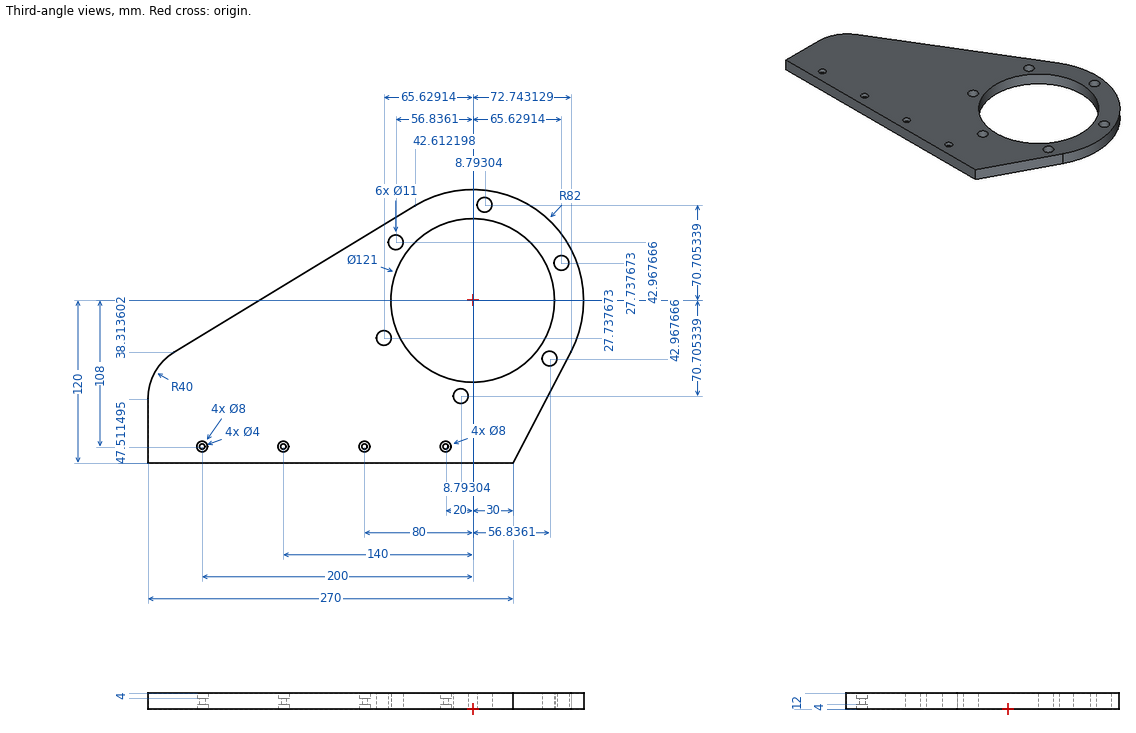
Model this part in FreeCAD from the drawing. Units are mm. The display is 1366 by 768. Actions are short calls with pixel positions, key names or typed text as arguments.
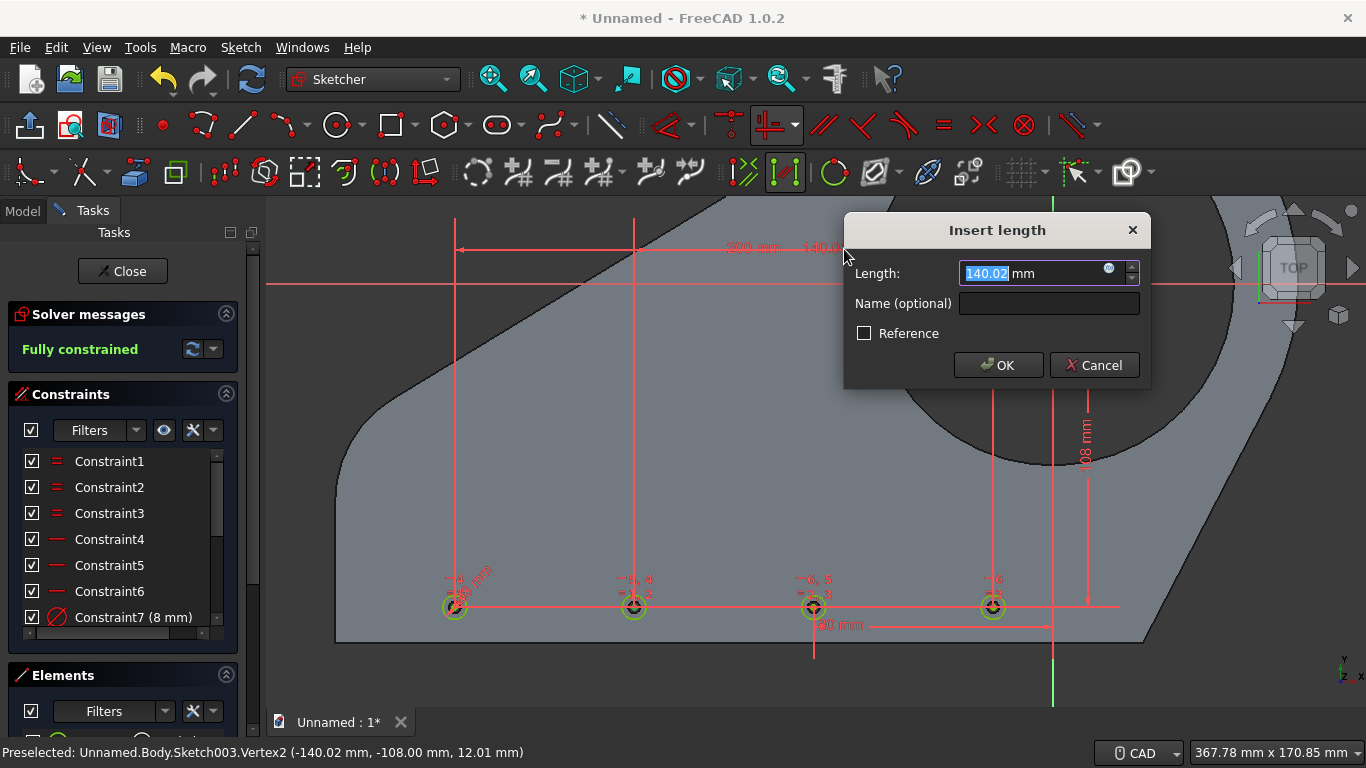
text(140)
key(Return)
key(Escape)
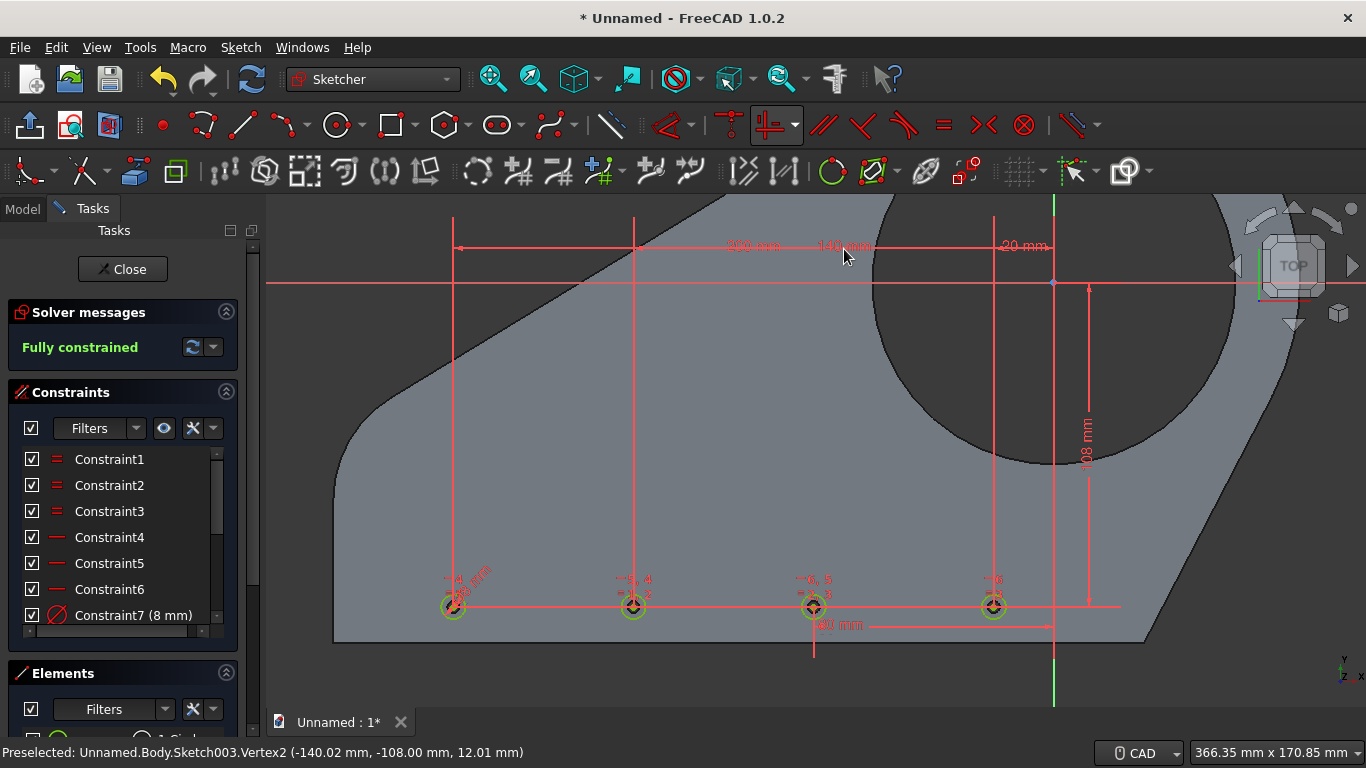
click(123, 269)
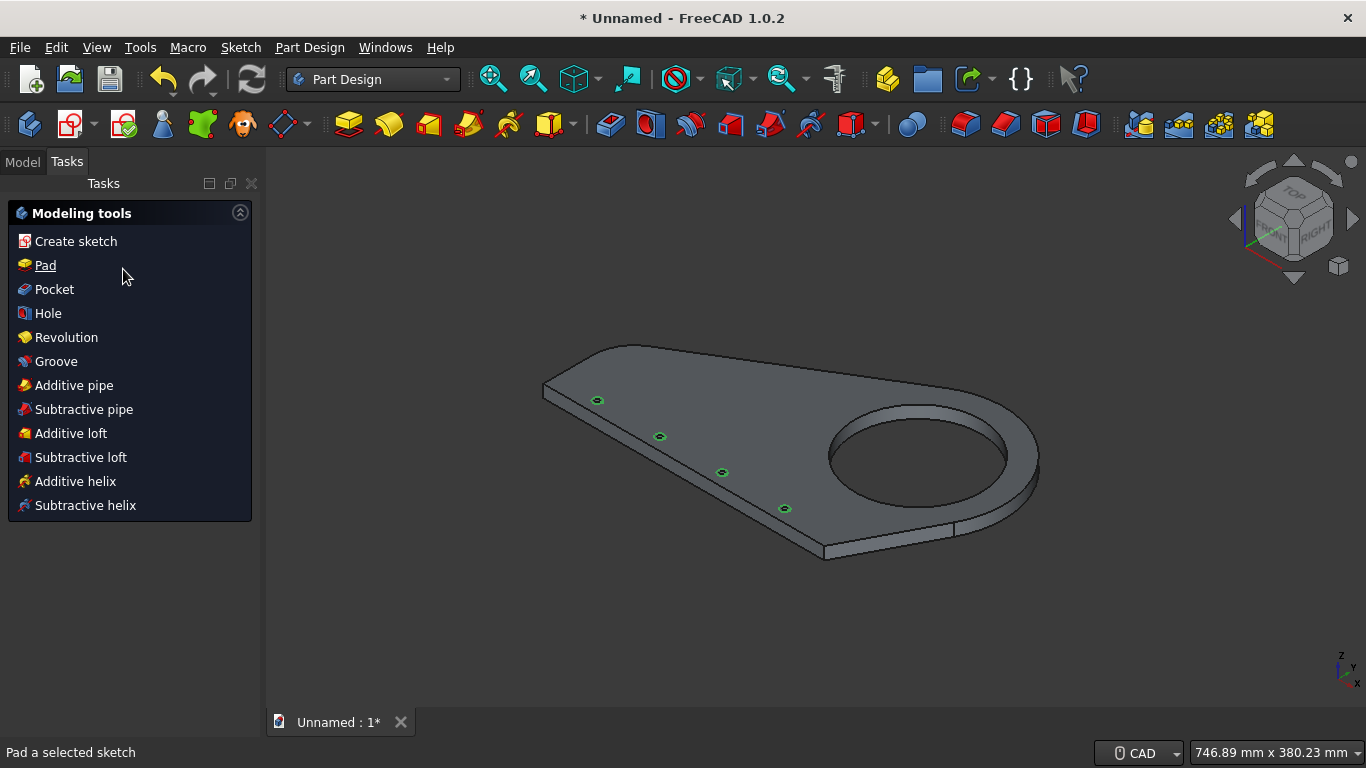
click(612, 124)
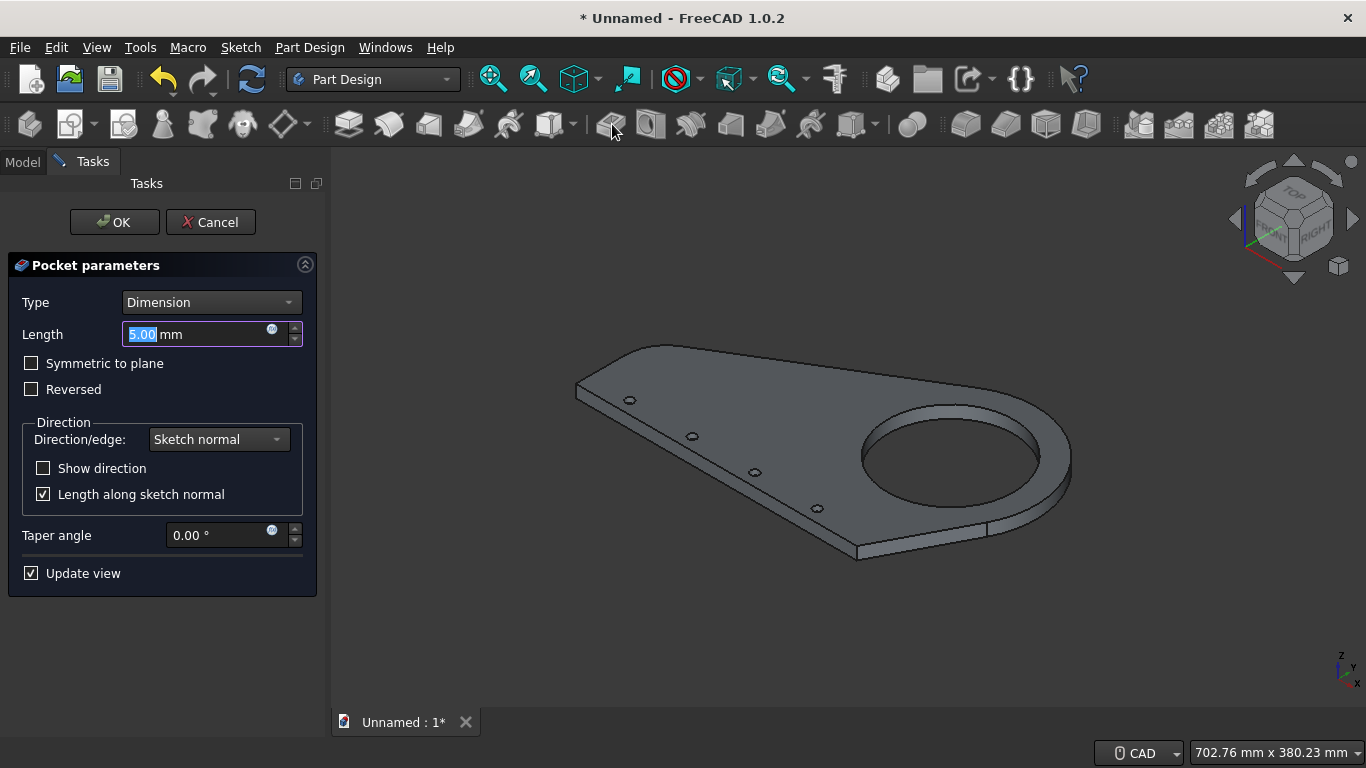
text(4)
key(Tab)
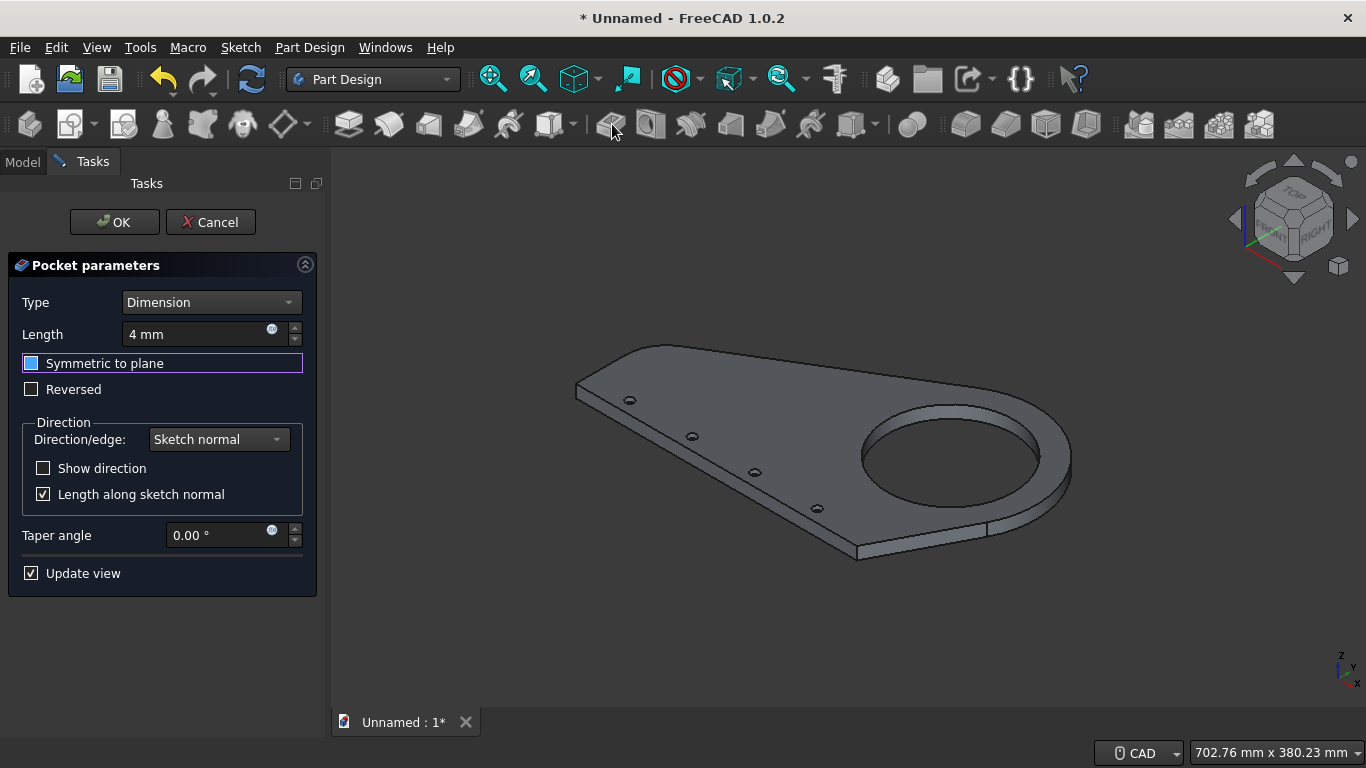
click(115, 222)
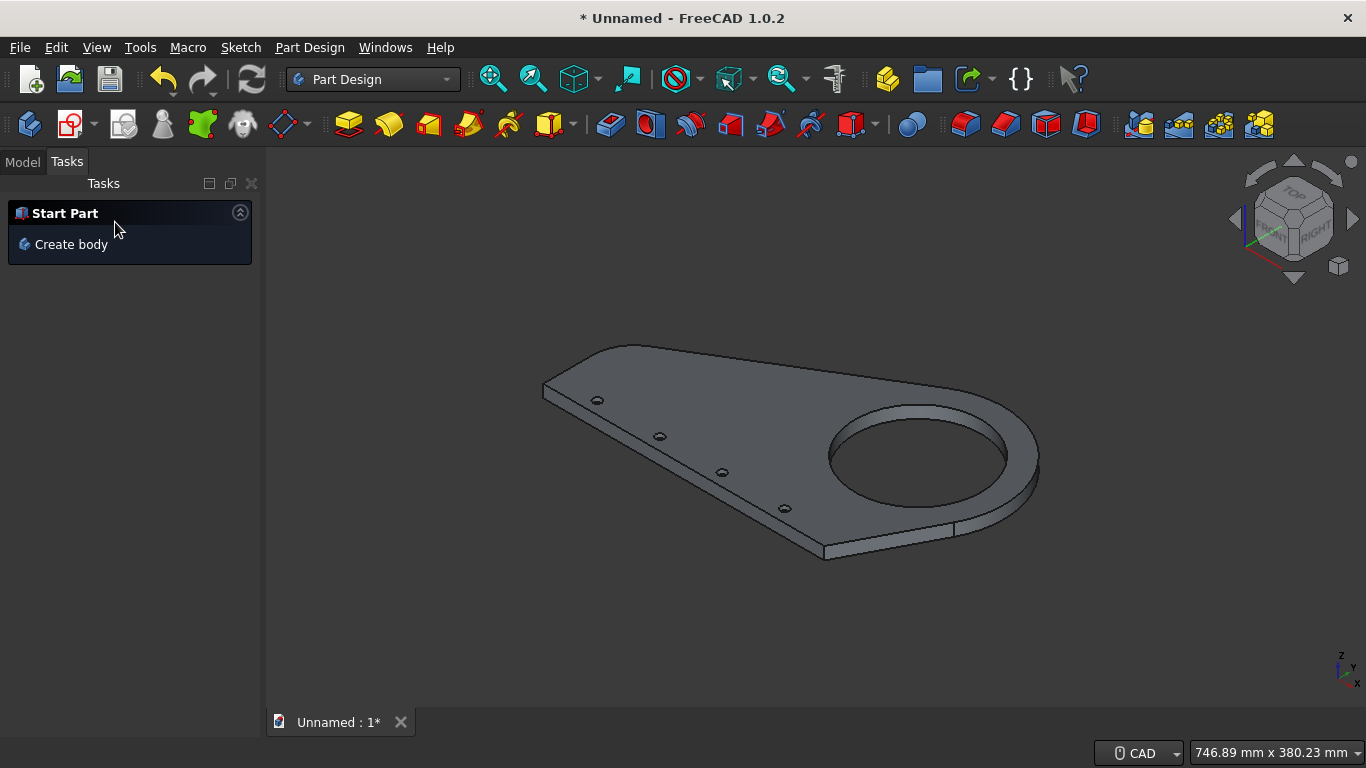
click(23, 161)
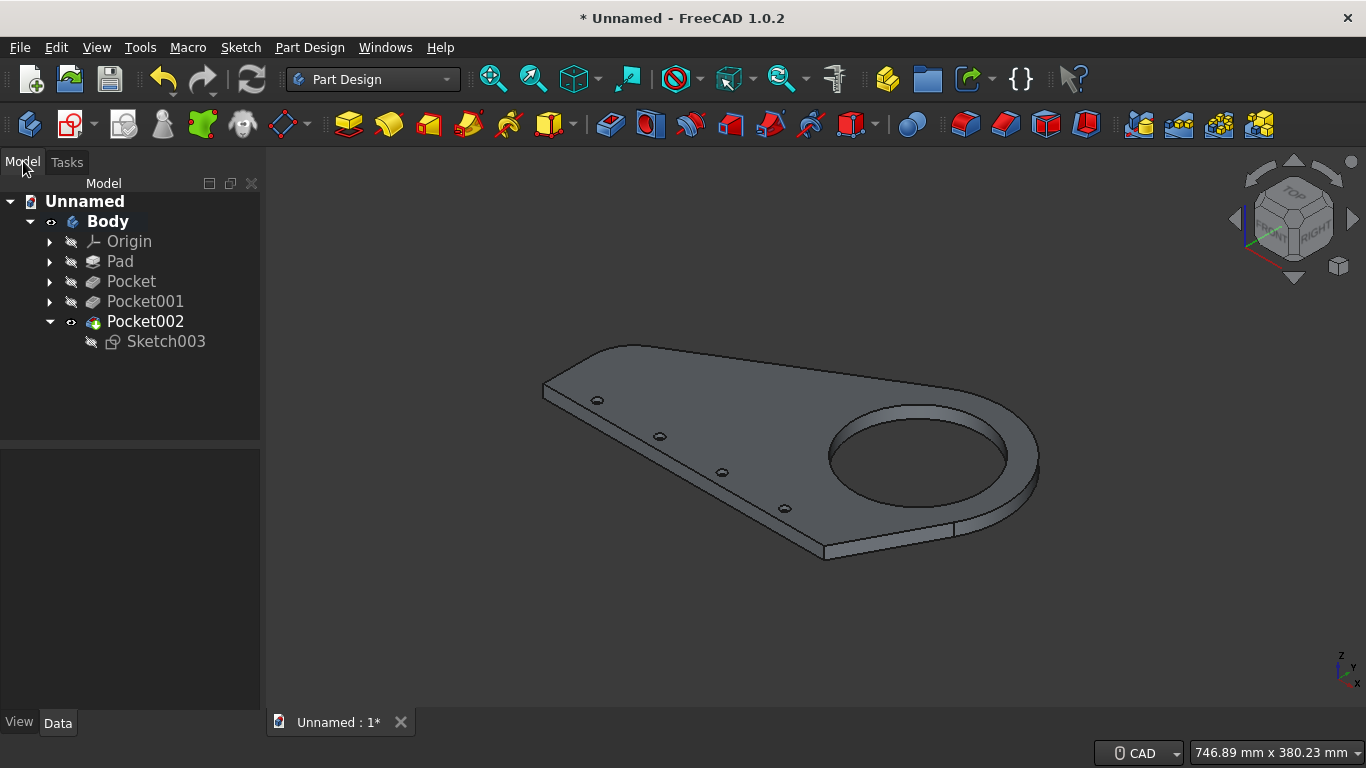
click(50, 242)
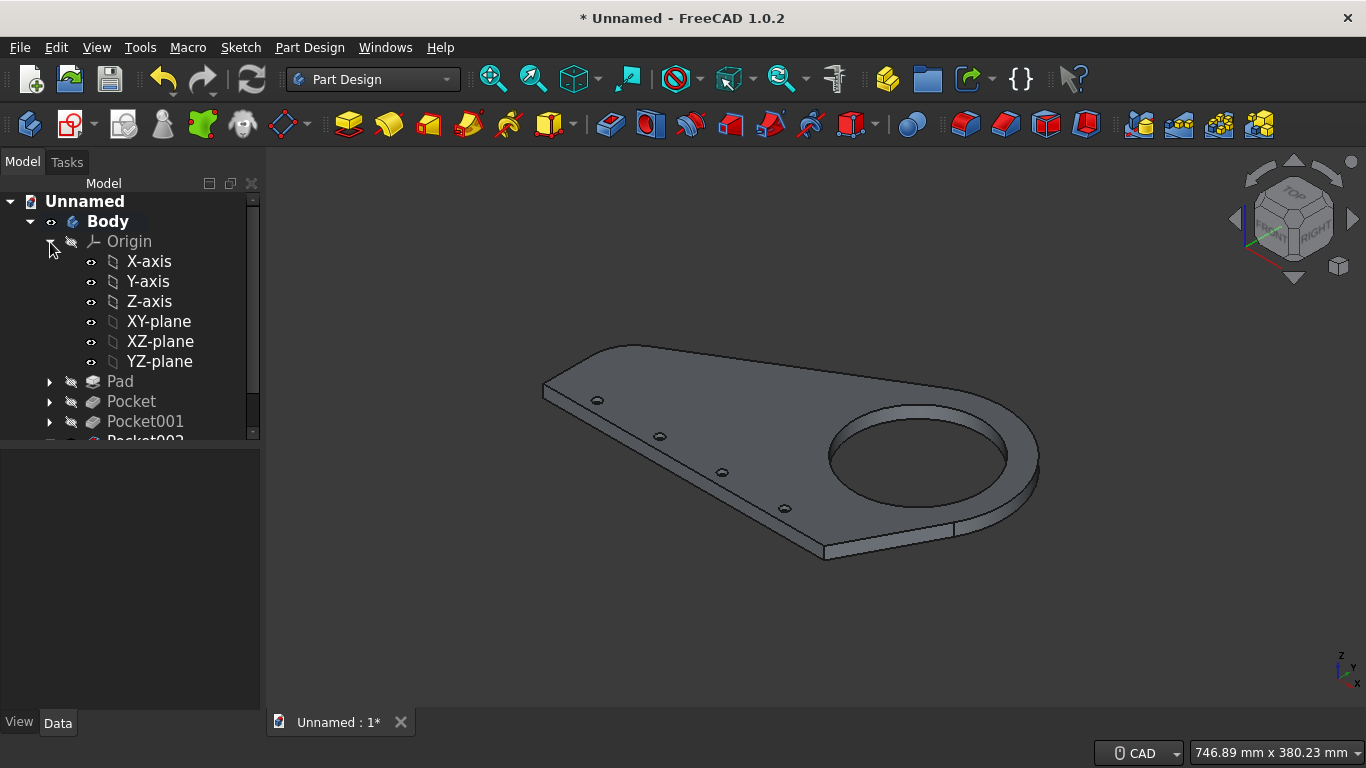
click(136, 322)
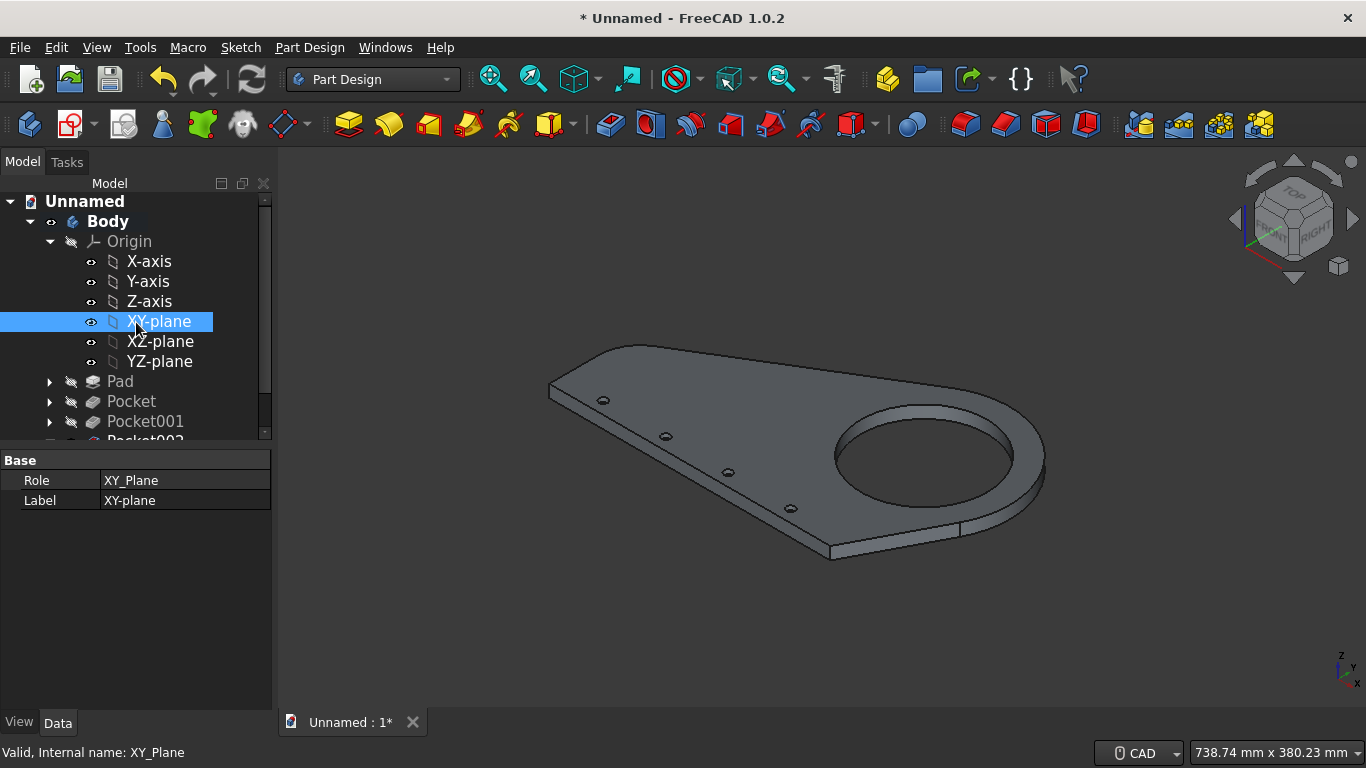
click(284, 124)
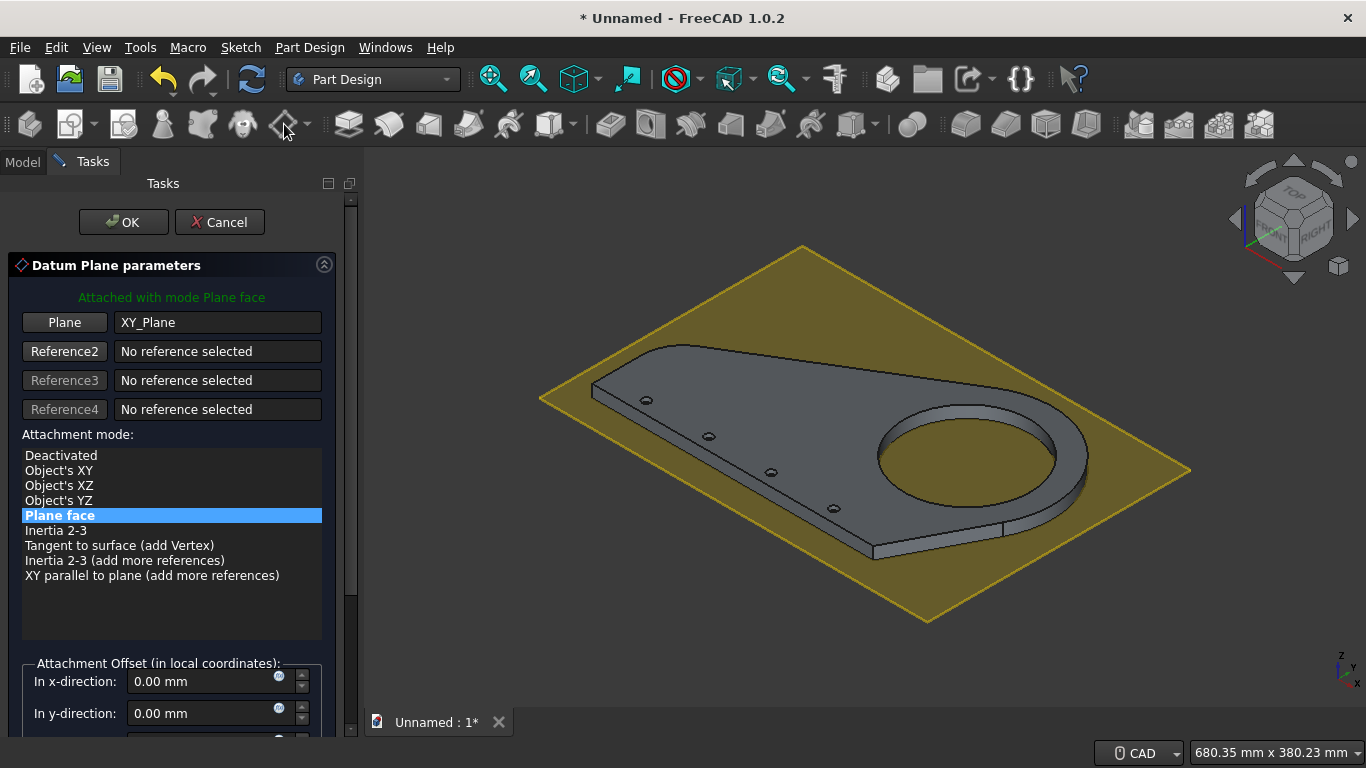
scroll(351, 464, down, 2)